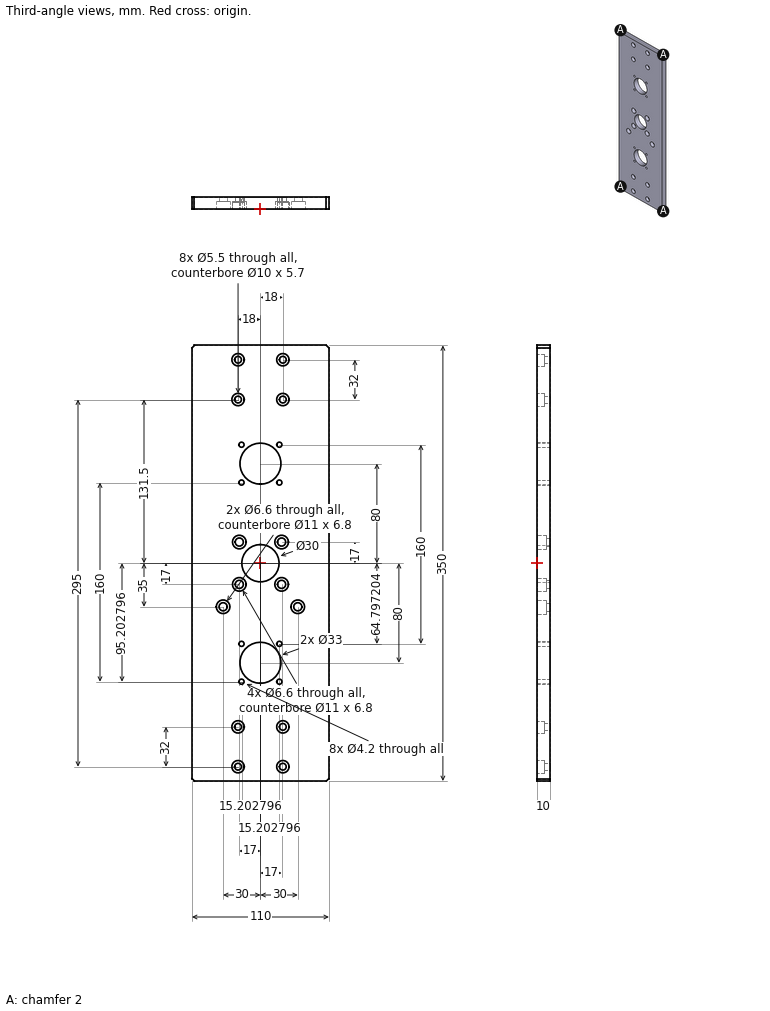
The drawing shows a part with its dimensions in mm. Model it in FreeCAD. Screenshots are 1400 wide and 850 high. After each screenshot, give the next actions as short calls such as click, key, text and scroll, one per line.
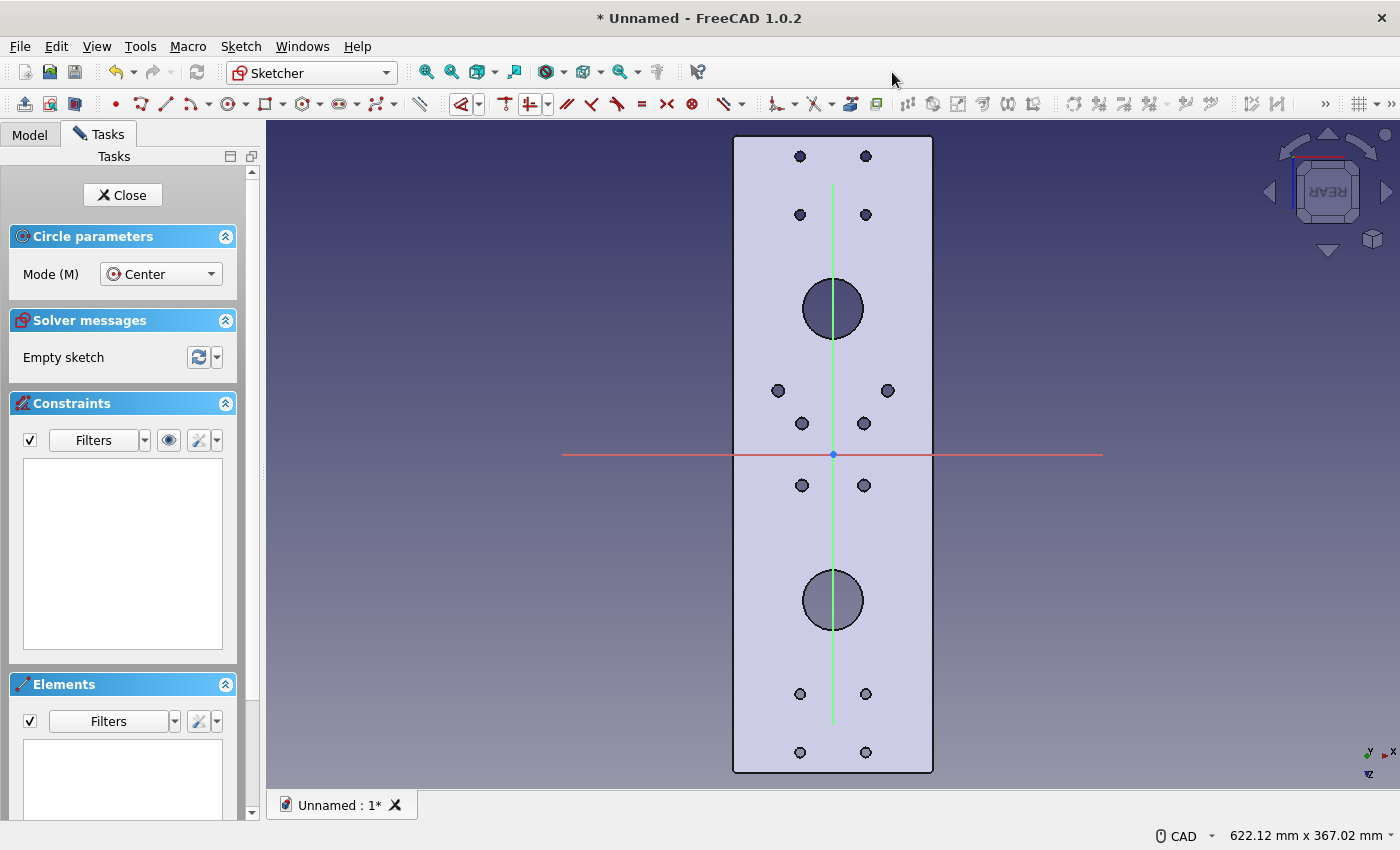
scroll(805, 281, up, 9)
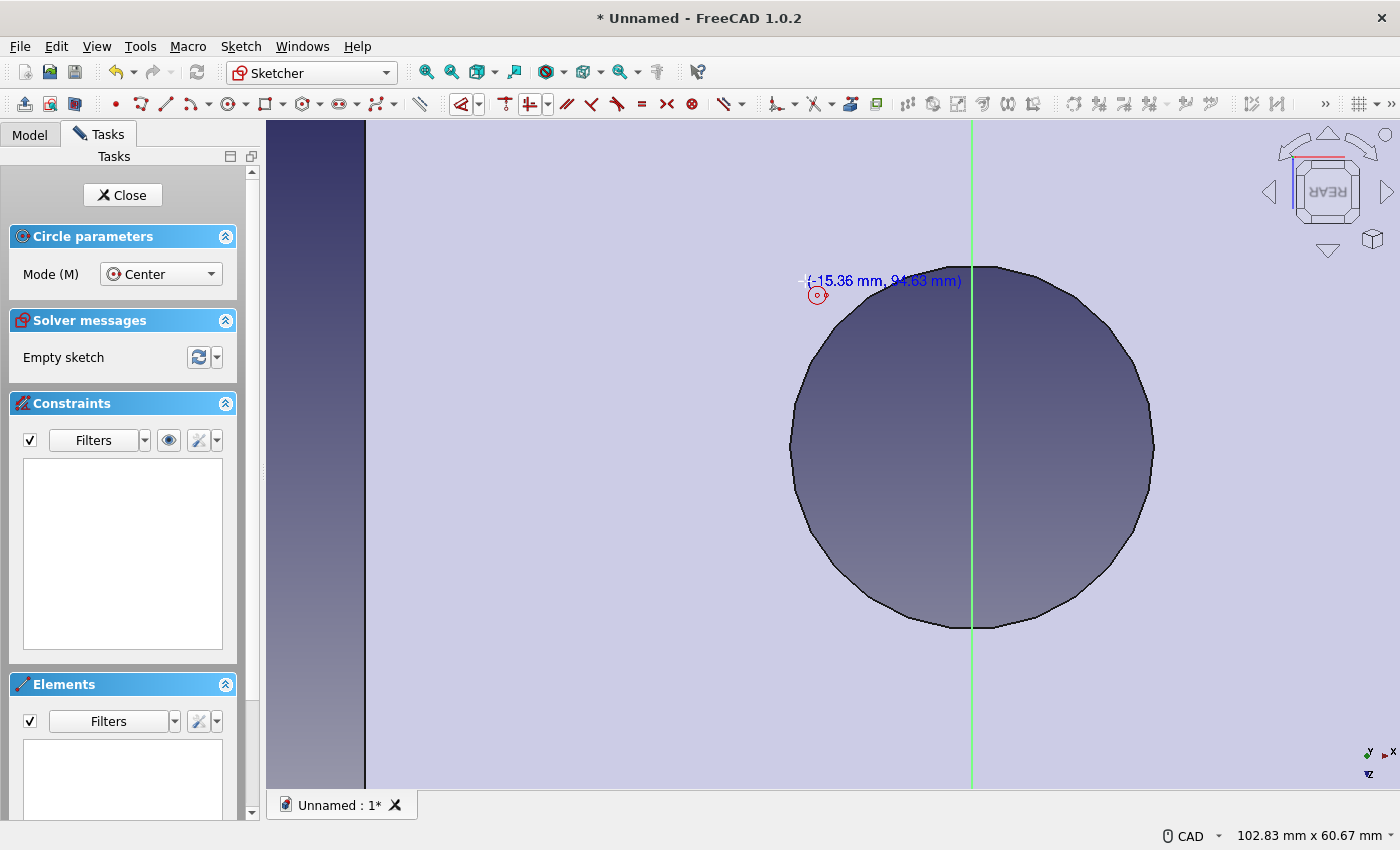
scroll(712, 233, down, 8)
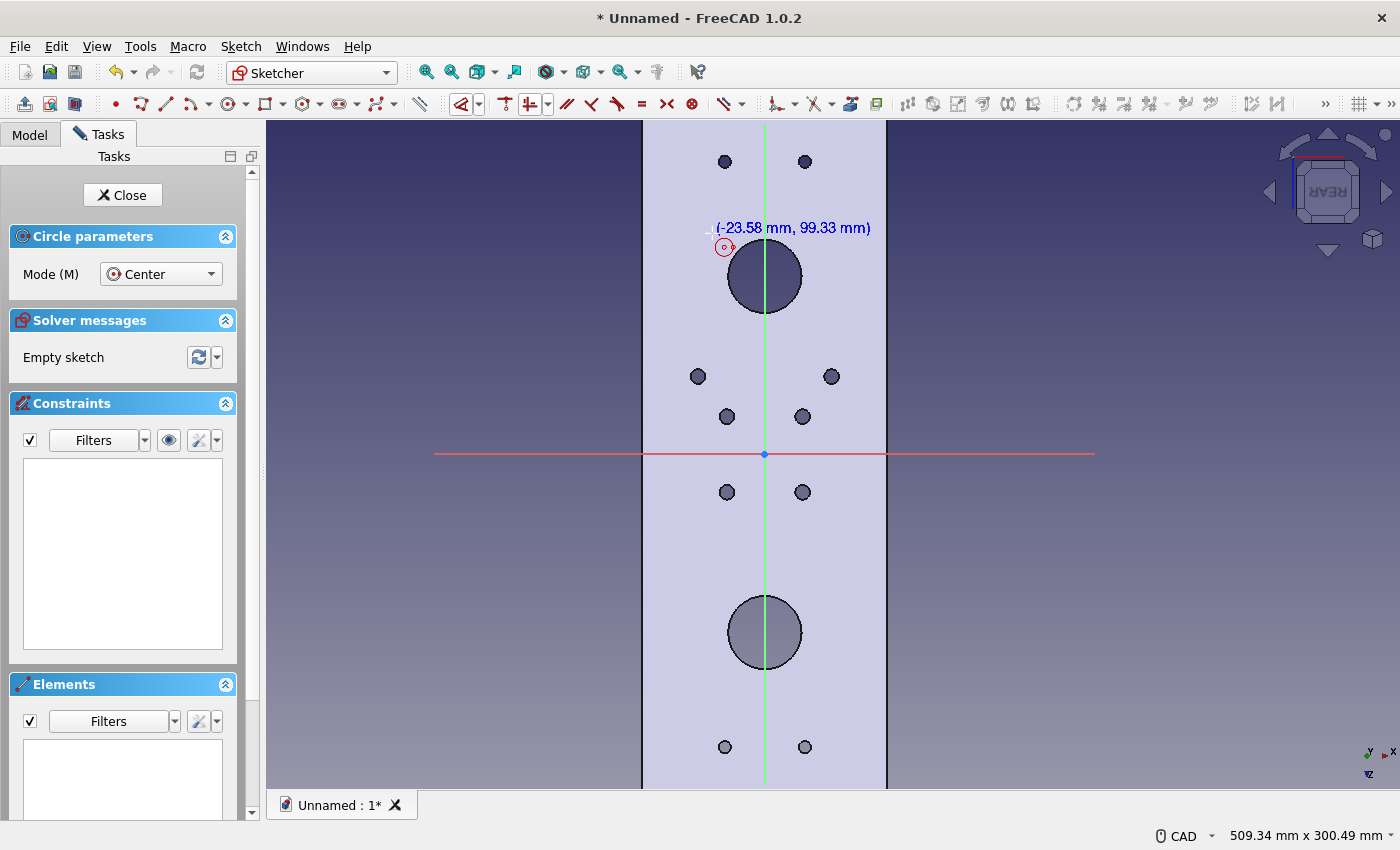
click(731, 243)
move(734, 239)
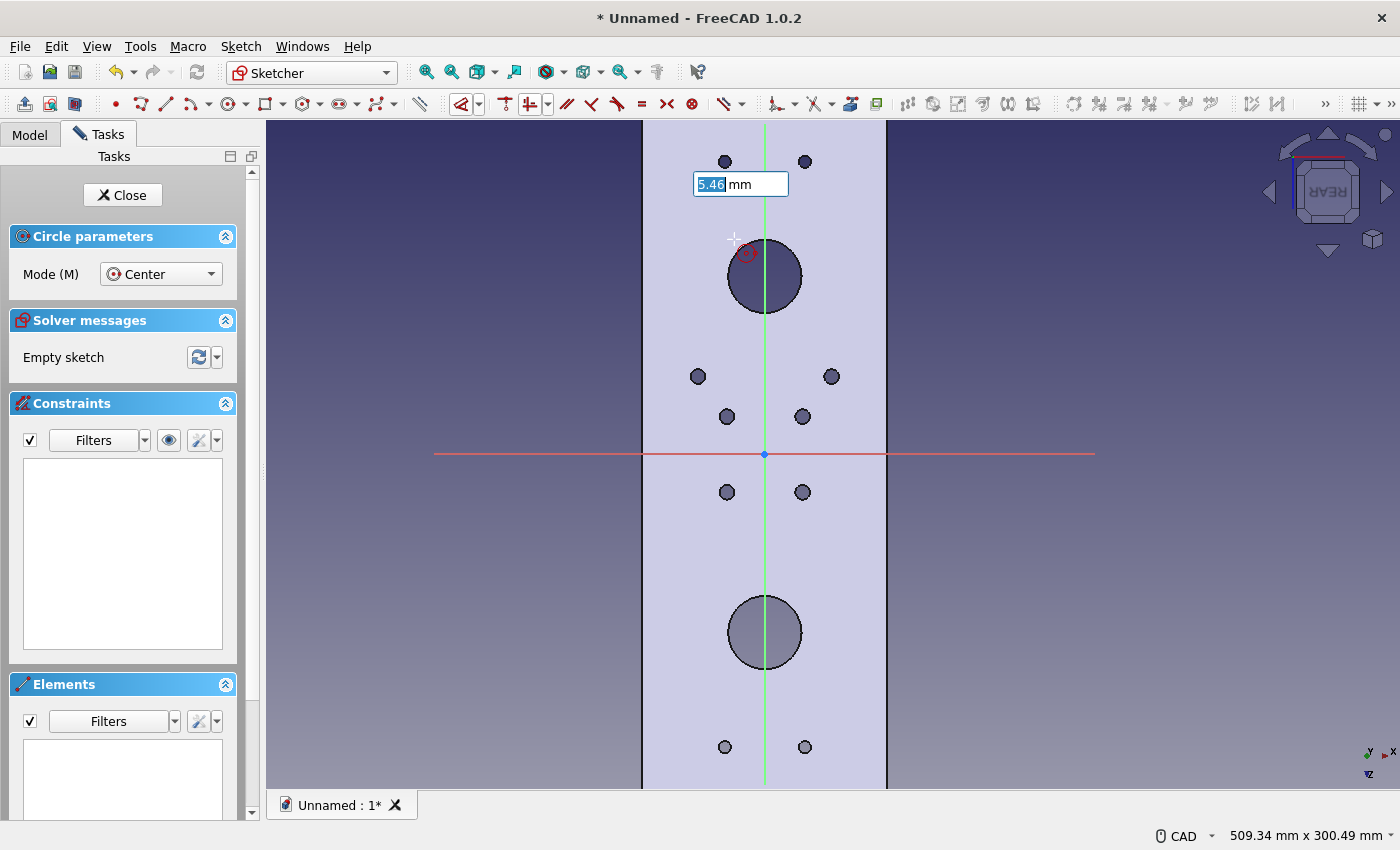
text(4.2)
key(Return)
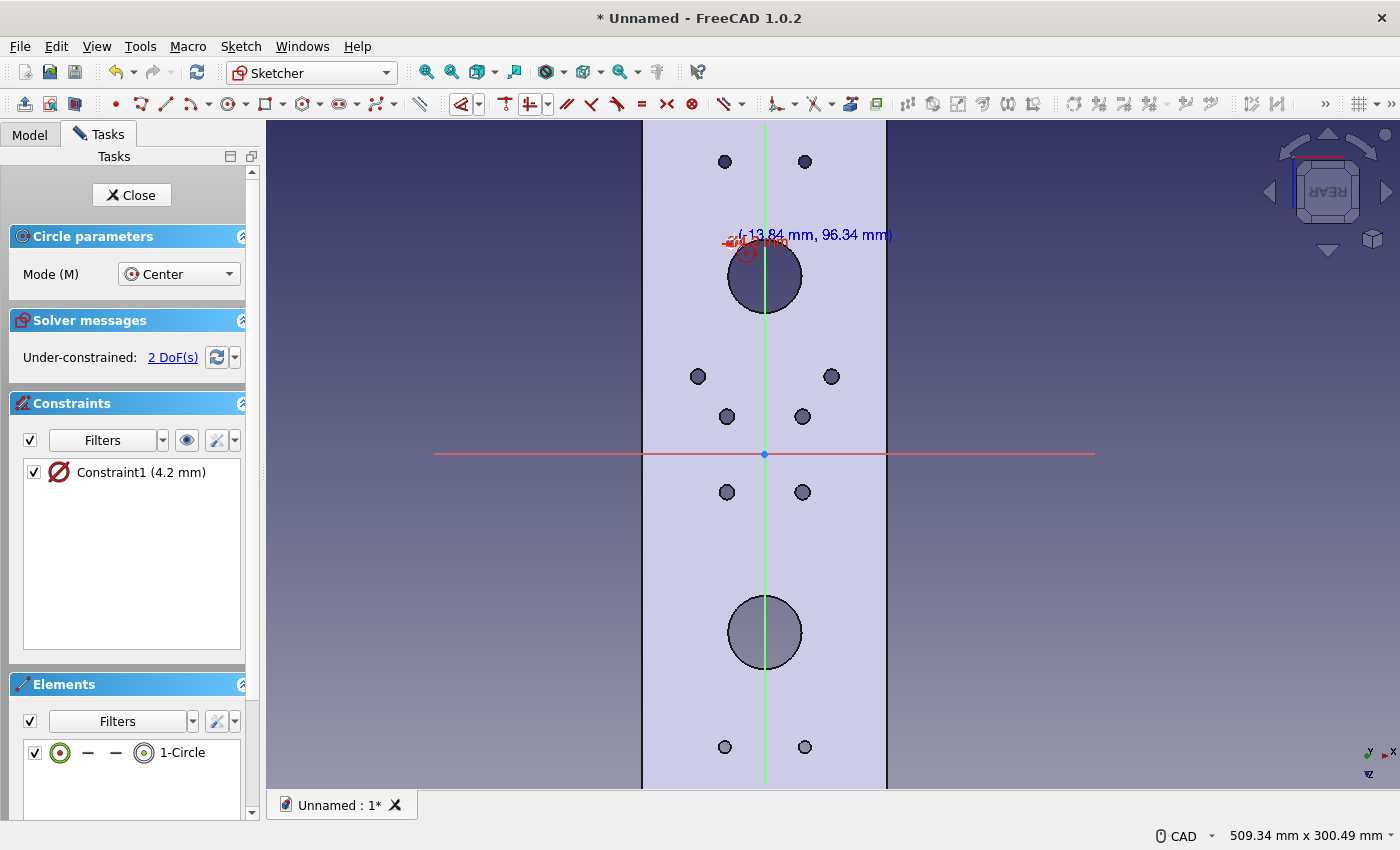
scroll(799, 310, up, 8)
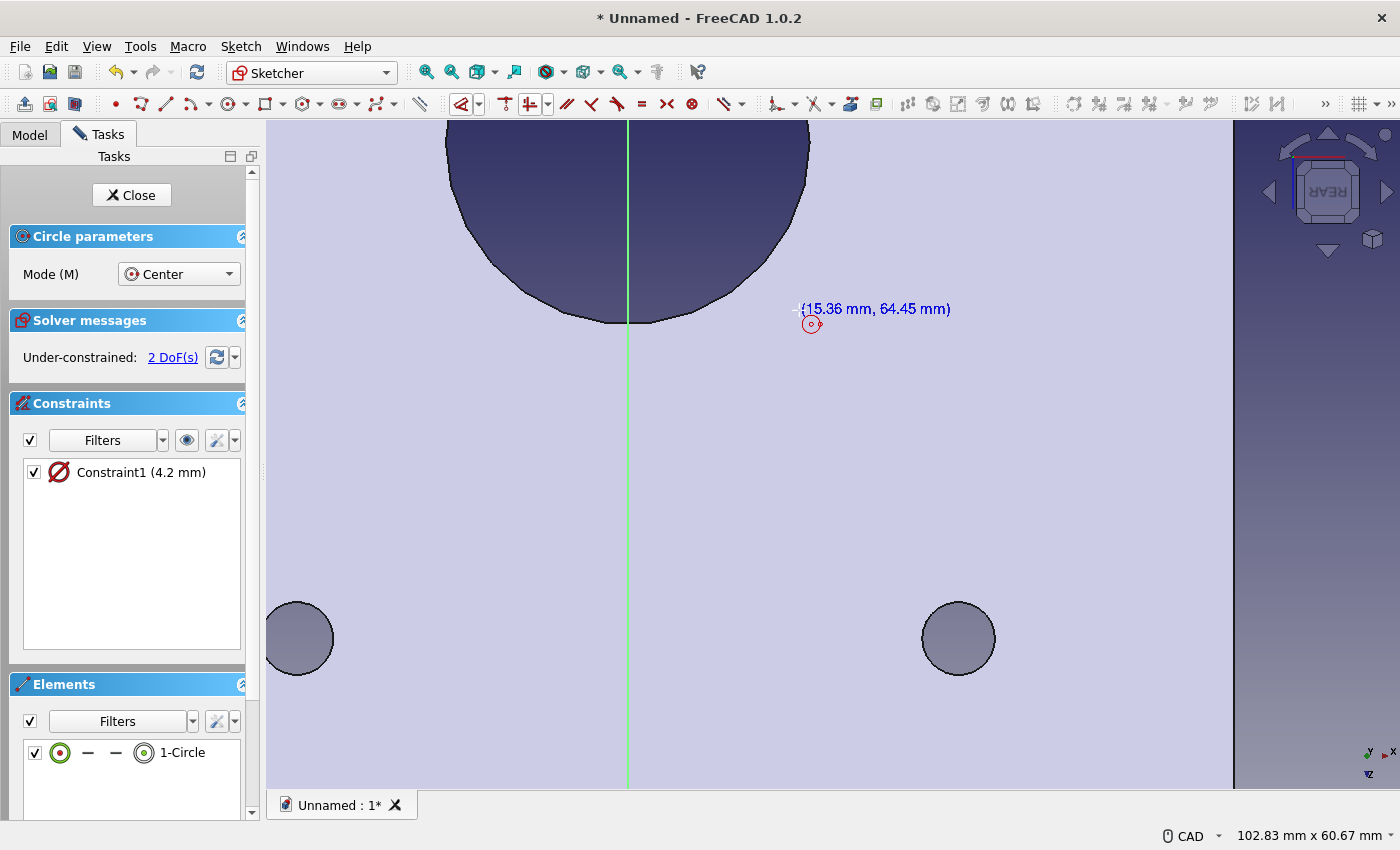
scroll(799, 310, down, 8)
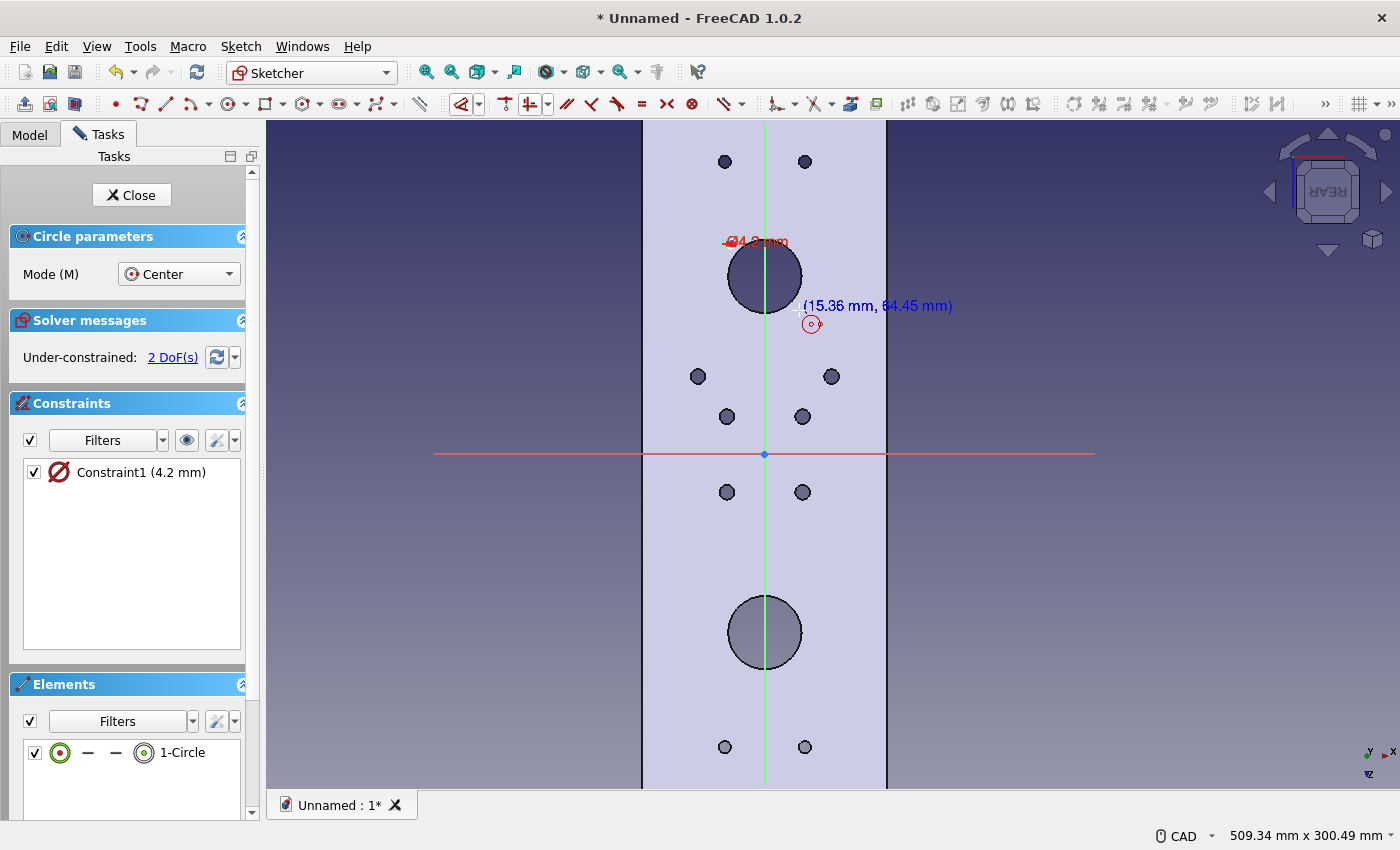
click(799, 310)
move(802, 307)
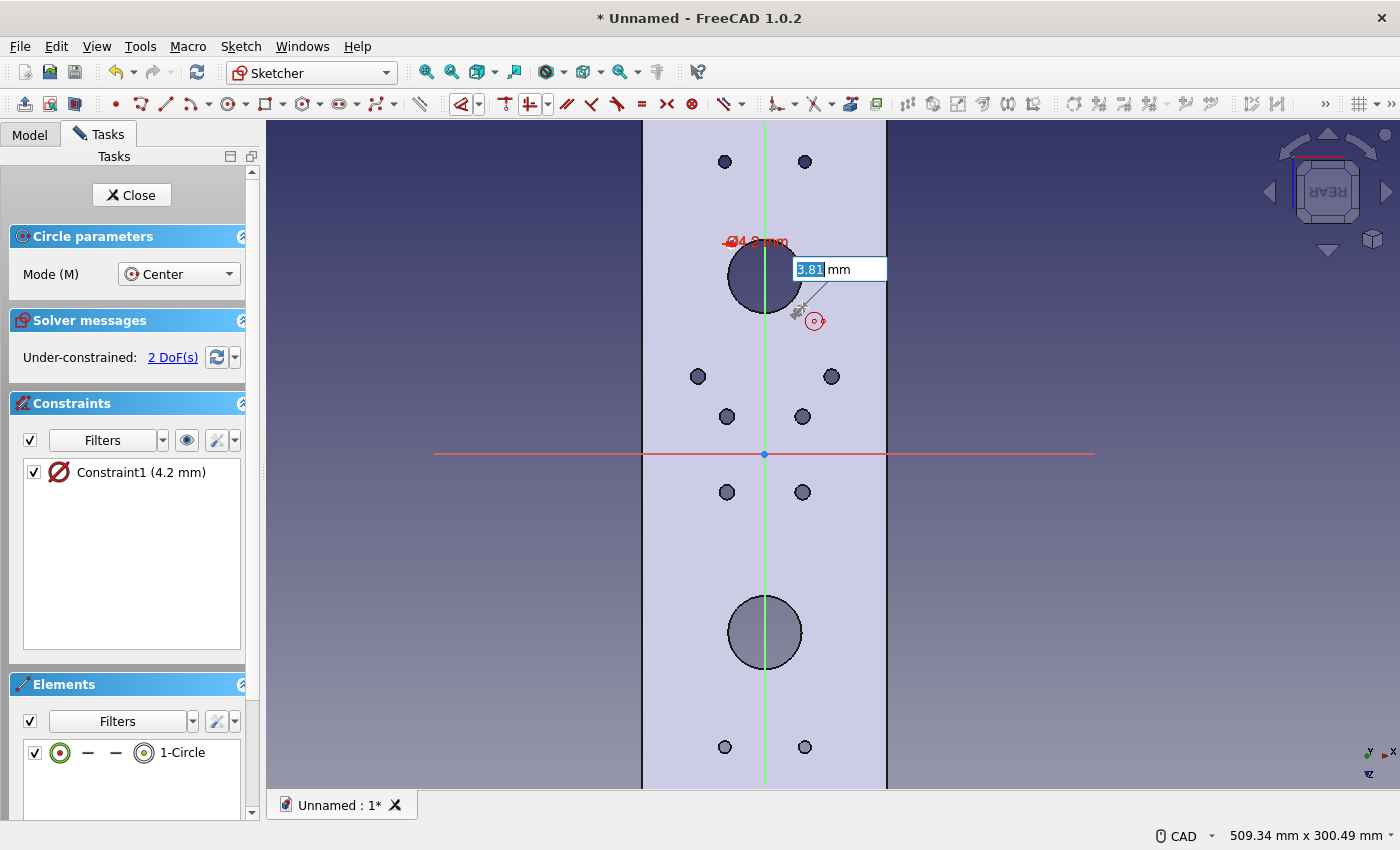
text(4.2)
key(Return)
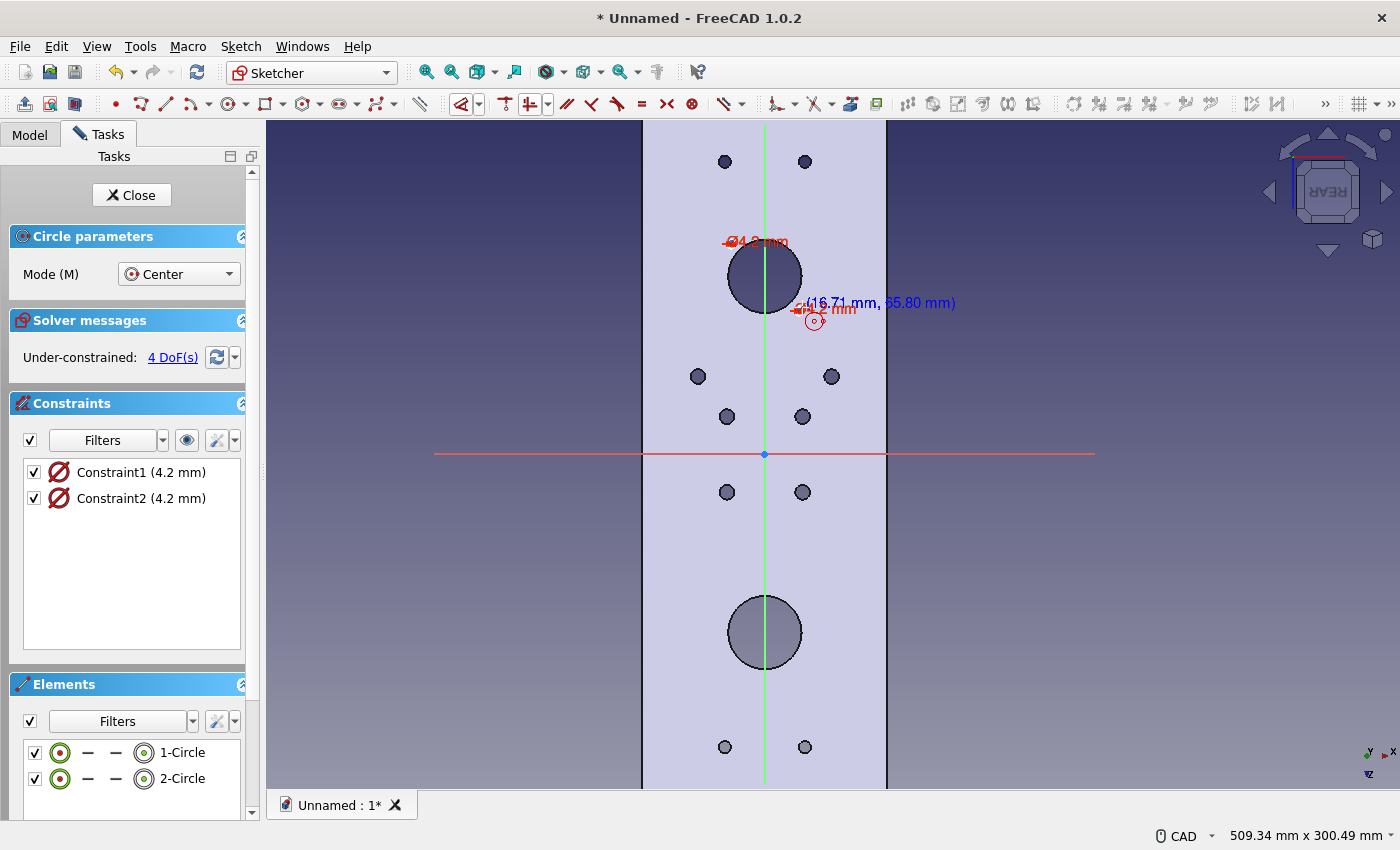
scroll(731, 310, up, 8)